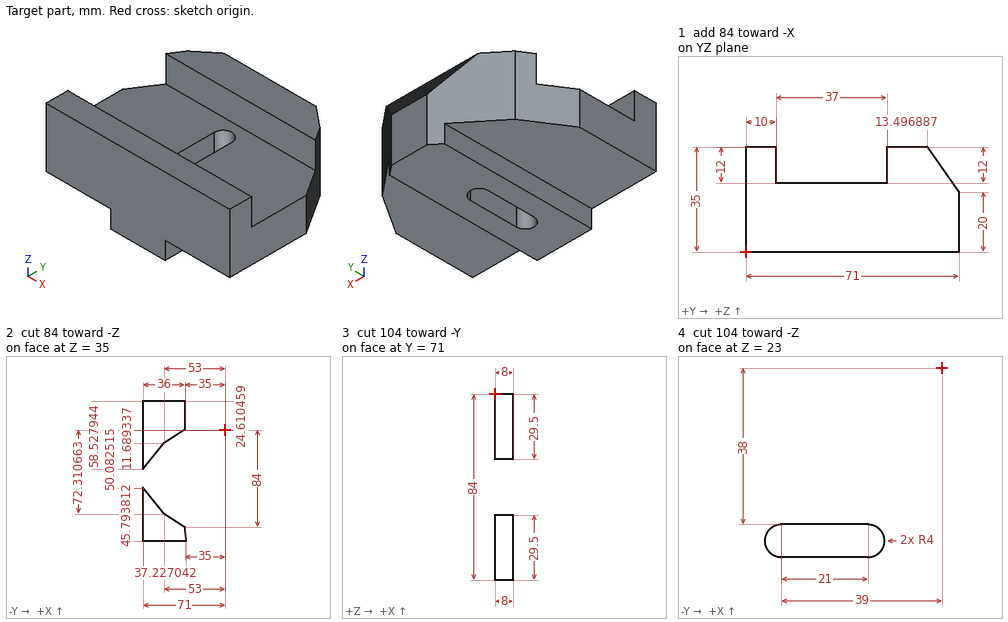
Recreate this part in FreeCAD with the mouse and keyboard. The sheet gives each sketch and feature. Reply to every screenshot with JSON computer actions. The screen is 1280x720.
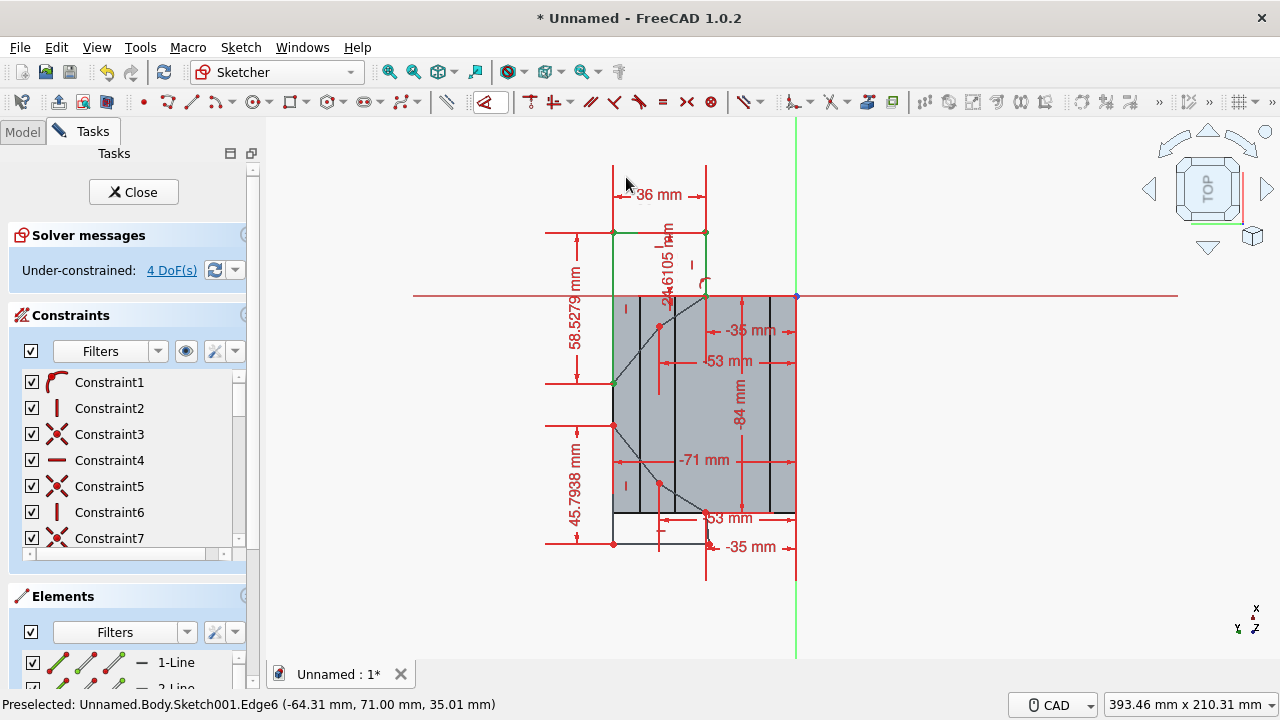
{"action": "left_click", "coordinate": [642, 544]}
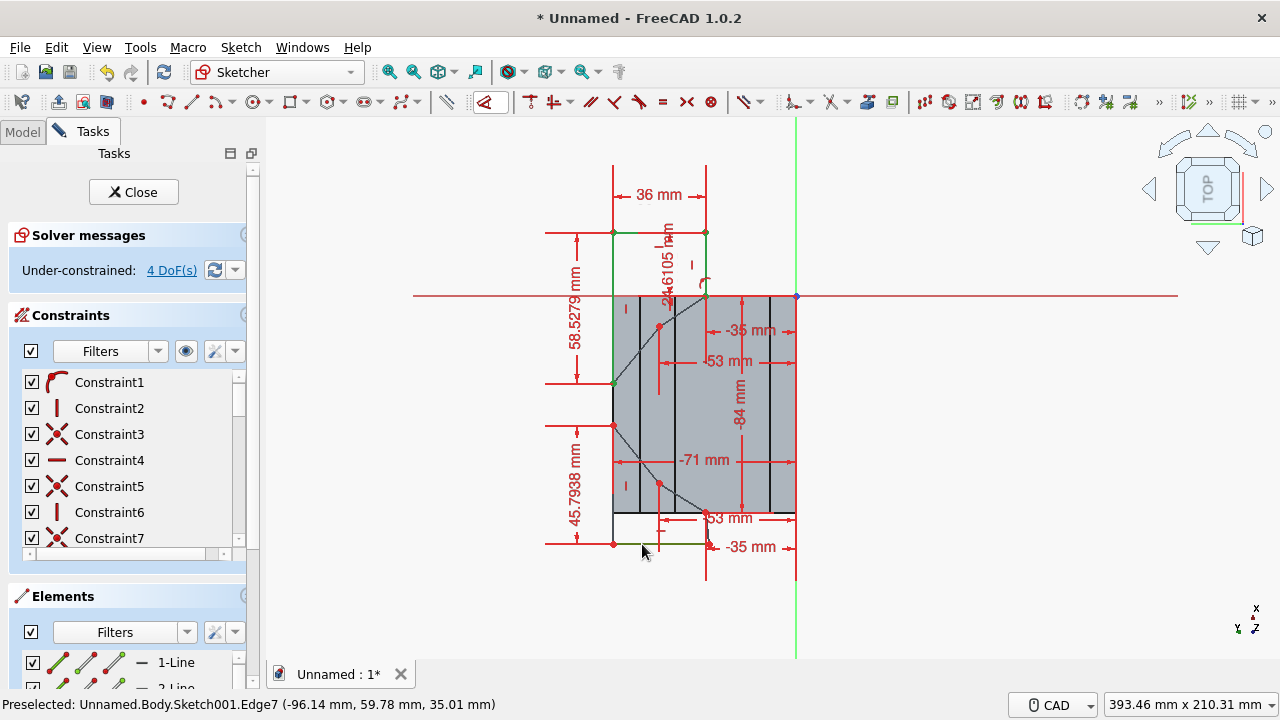
{"action": "left_click", "coordinate": [502, 102]}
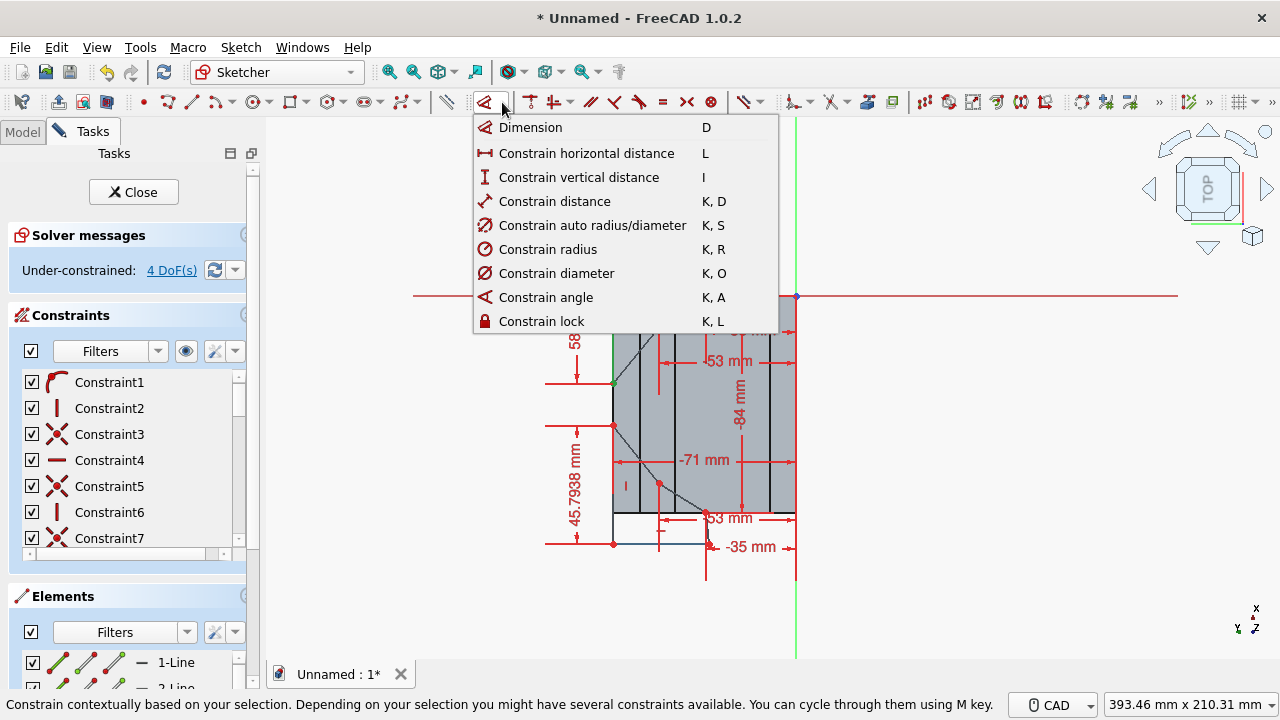
{"action": "left_click", "coordinate": [626, 153]}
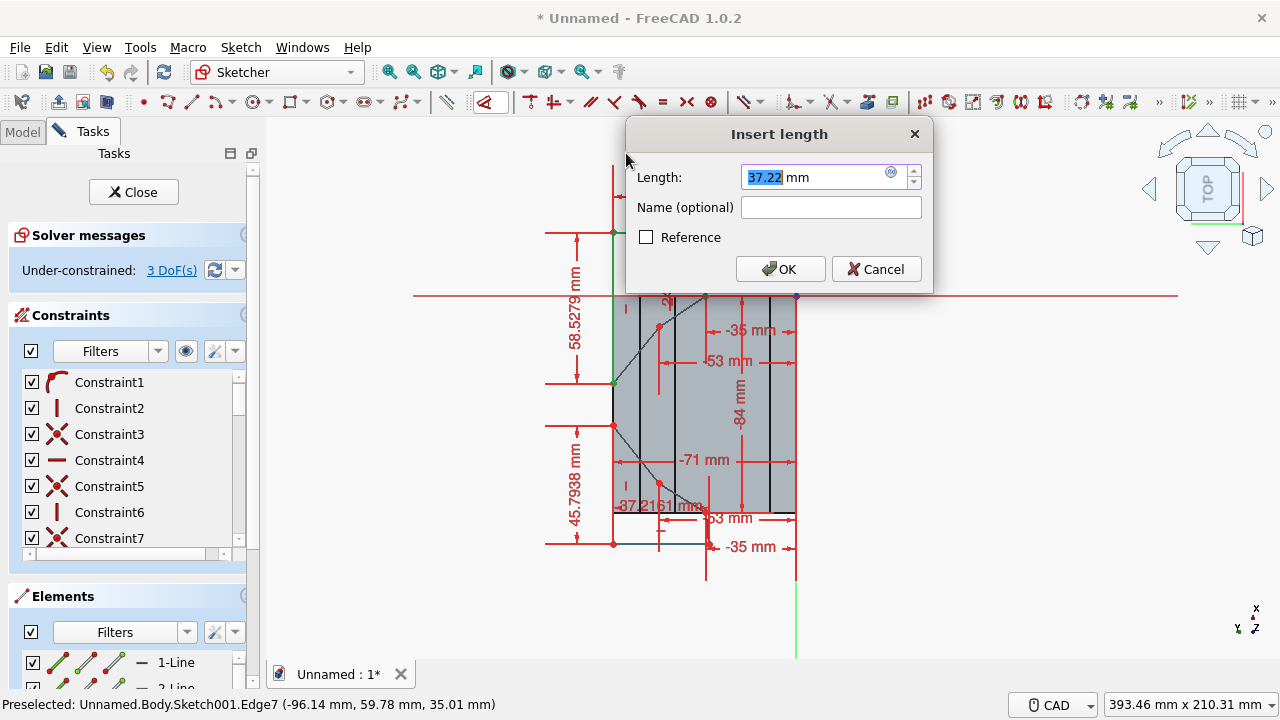
{"action": "type", "text": "37.227042"}
{"action": "key", "text": "Return"}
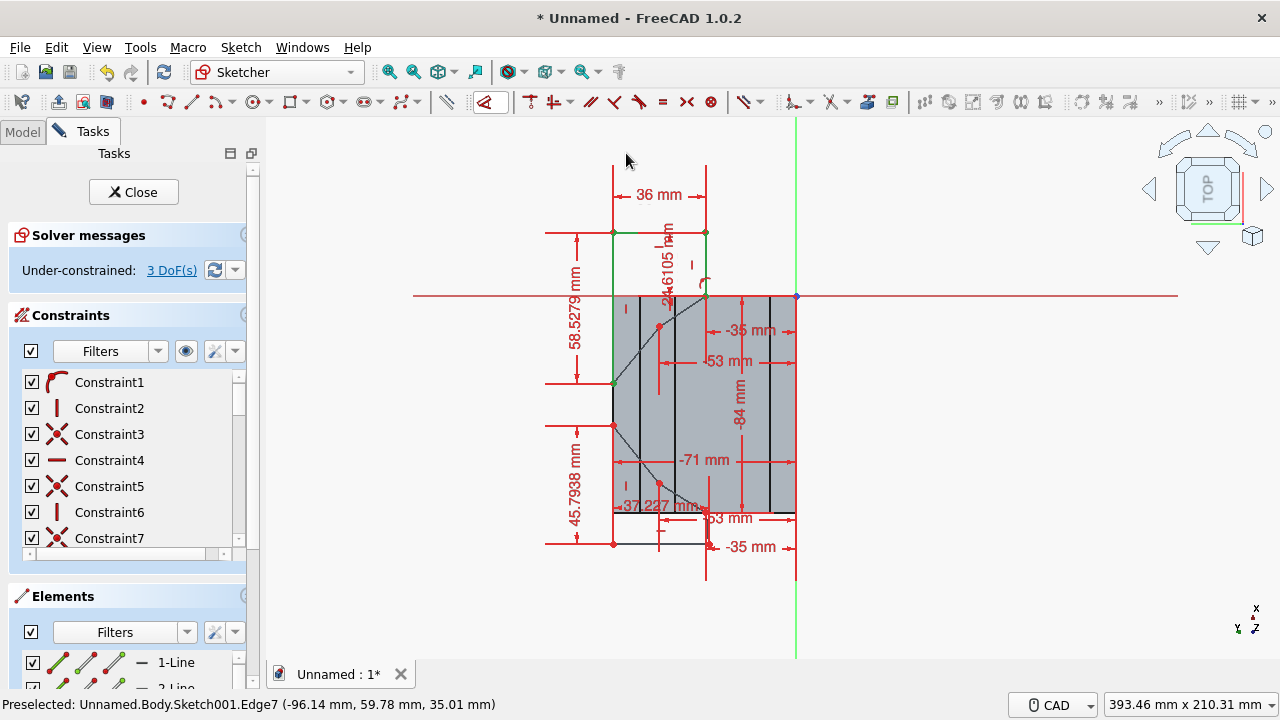
{"action": "scroll", "coordinate": [659, 327], "scroll_direction": "up", "scroll_amount": 2}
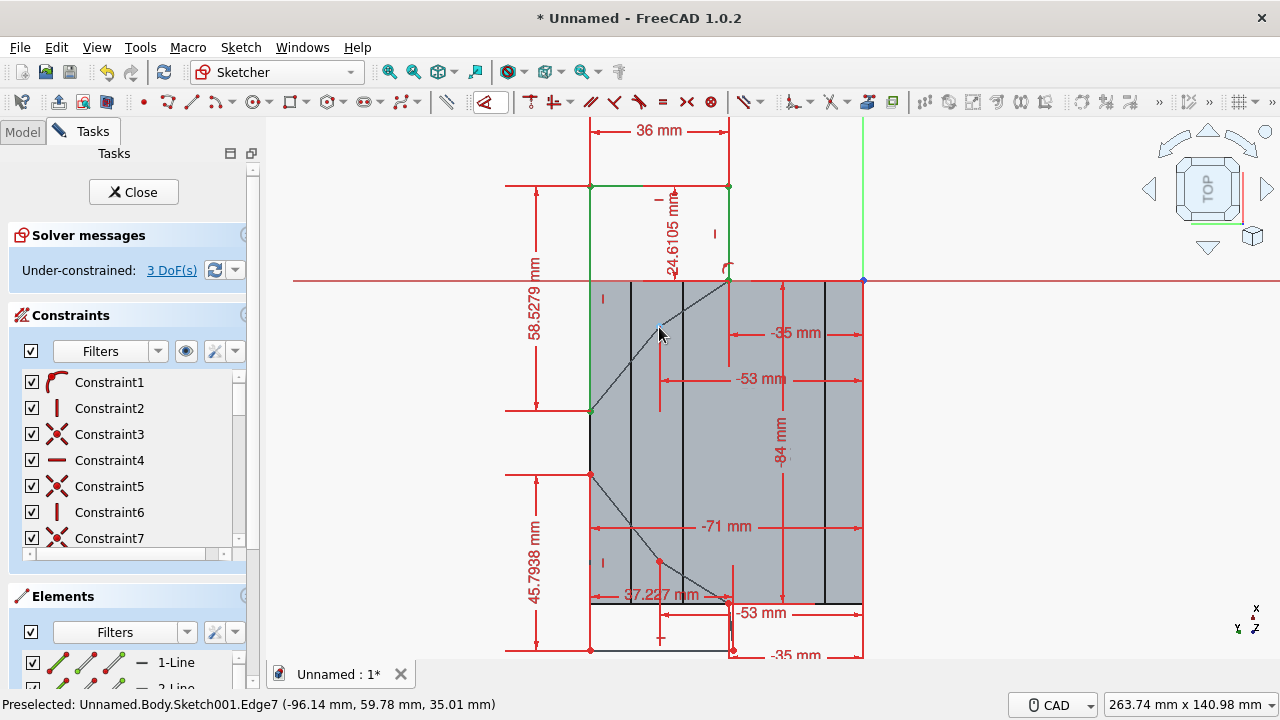
{"action": "left_click", "coordinate": [660, 327]}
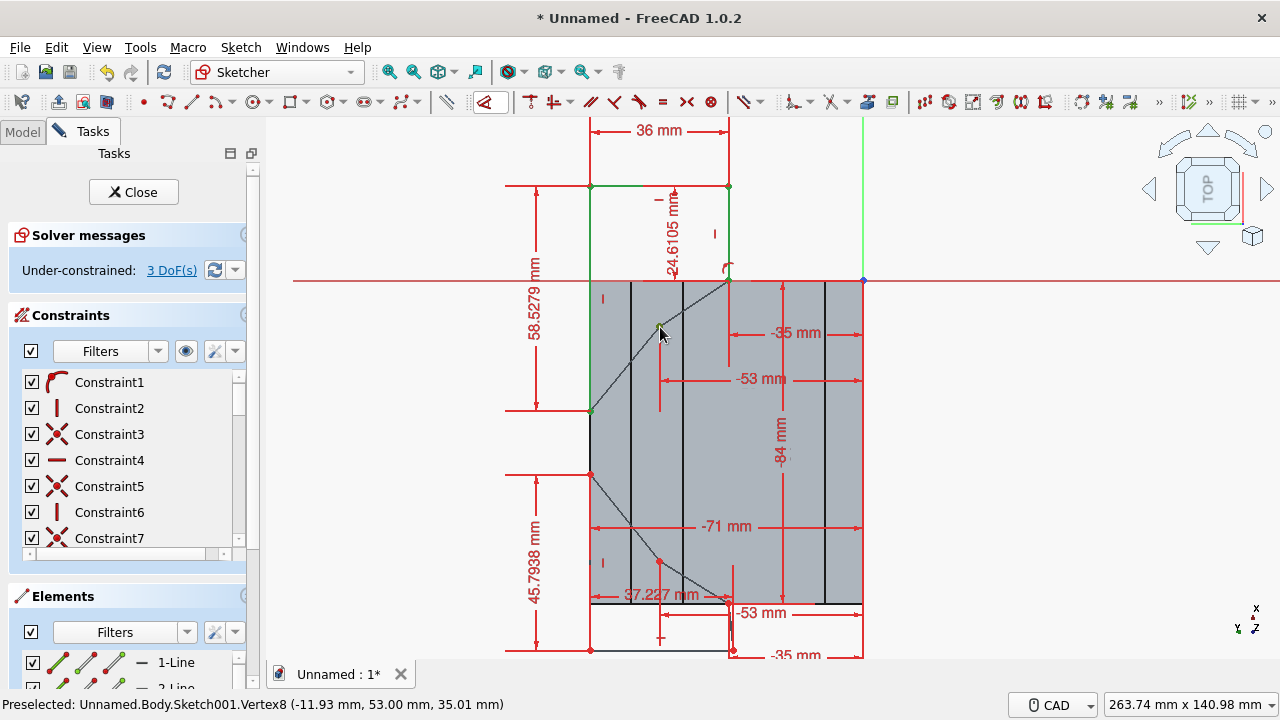
{"action": "left_click", "coordinate": [502, 102]}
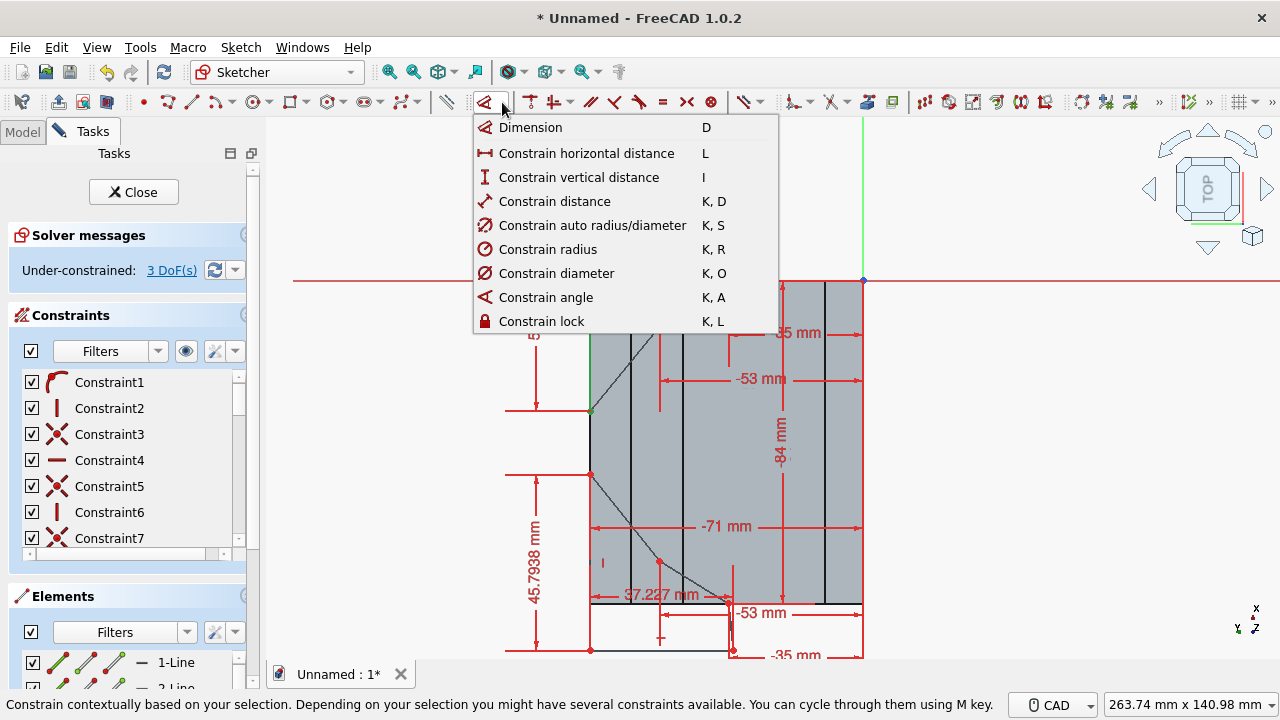
{"action": "left_click", "coordinate": [626, 177]}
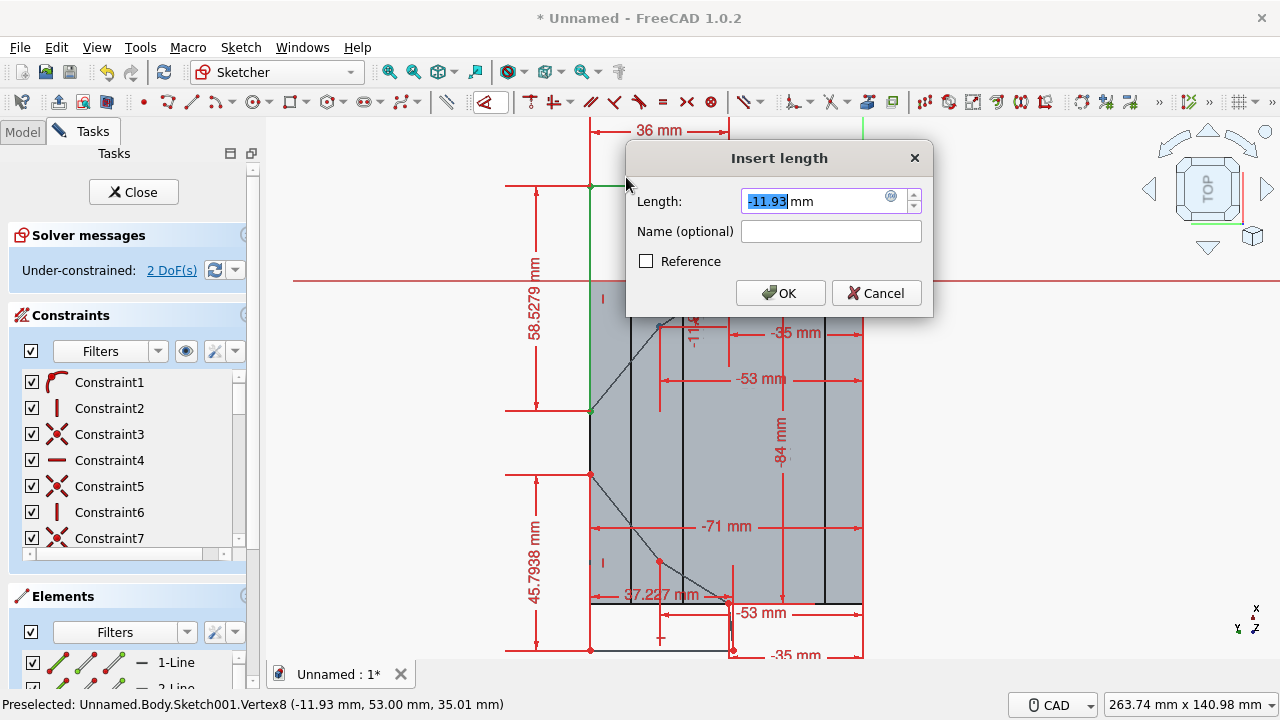
{"action": "type", "text": "-11.689337"}
{"action": "key", "text": "Return"}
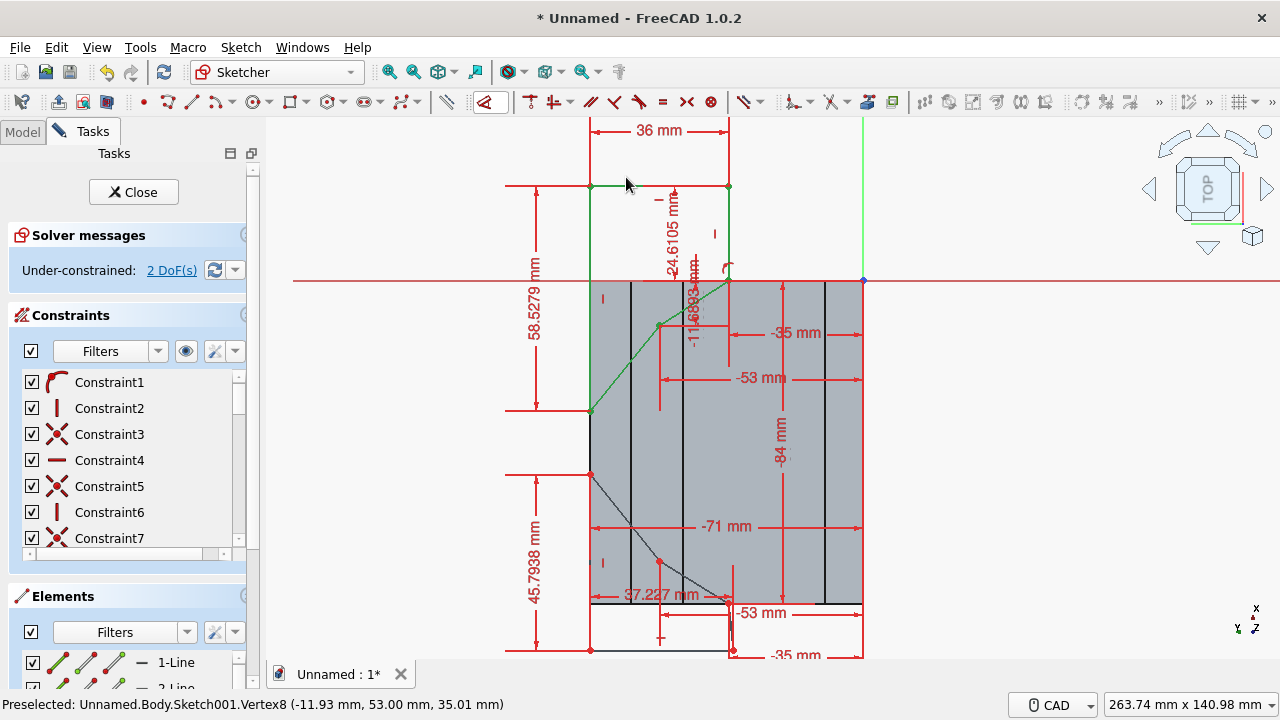
{"action": "left_click", "coordinate": [590, 474]}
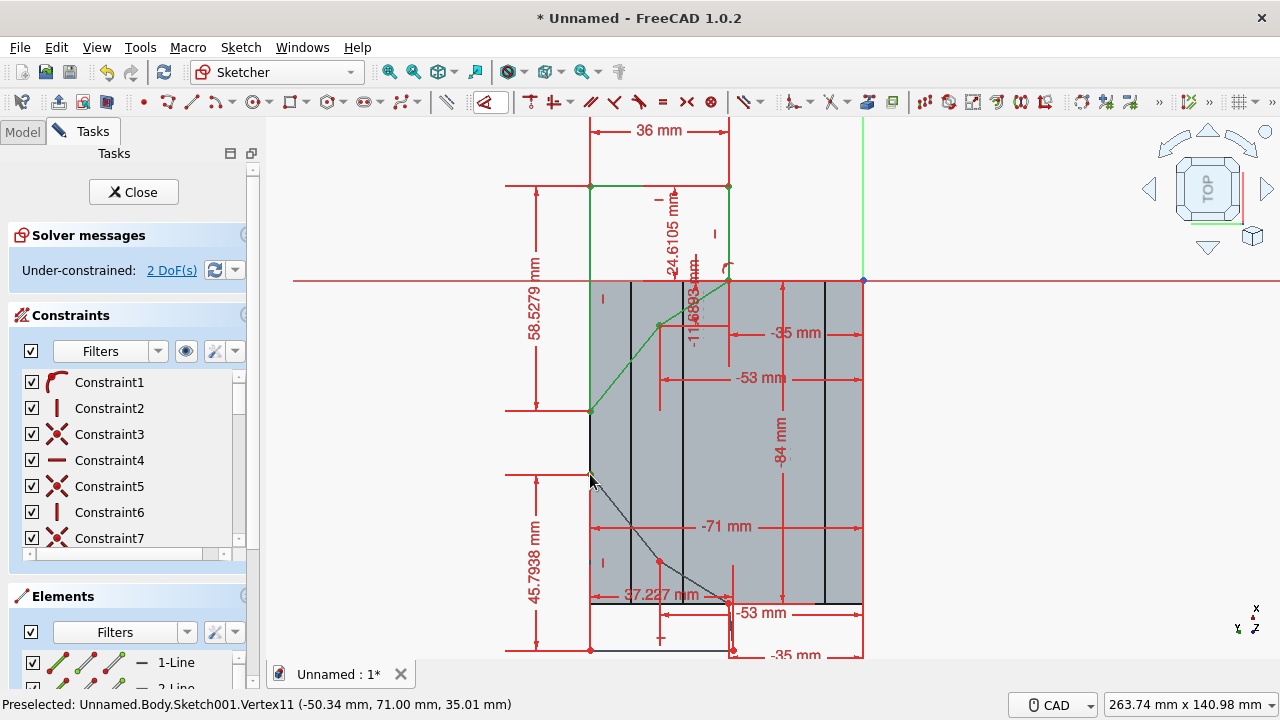
{"action": "left_click", "coordinate": [502, 102]}